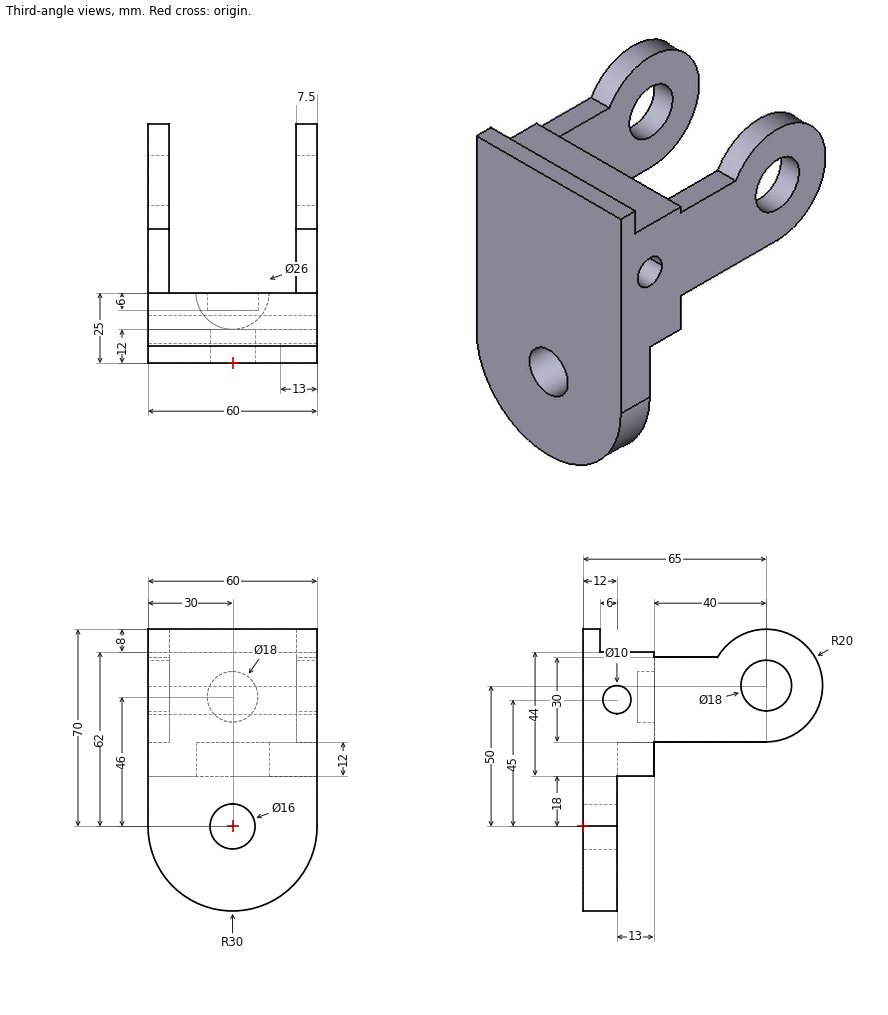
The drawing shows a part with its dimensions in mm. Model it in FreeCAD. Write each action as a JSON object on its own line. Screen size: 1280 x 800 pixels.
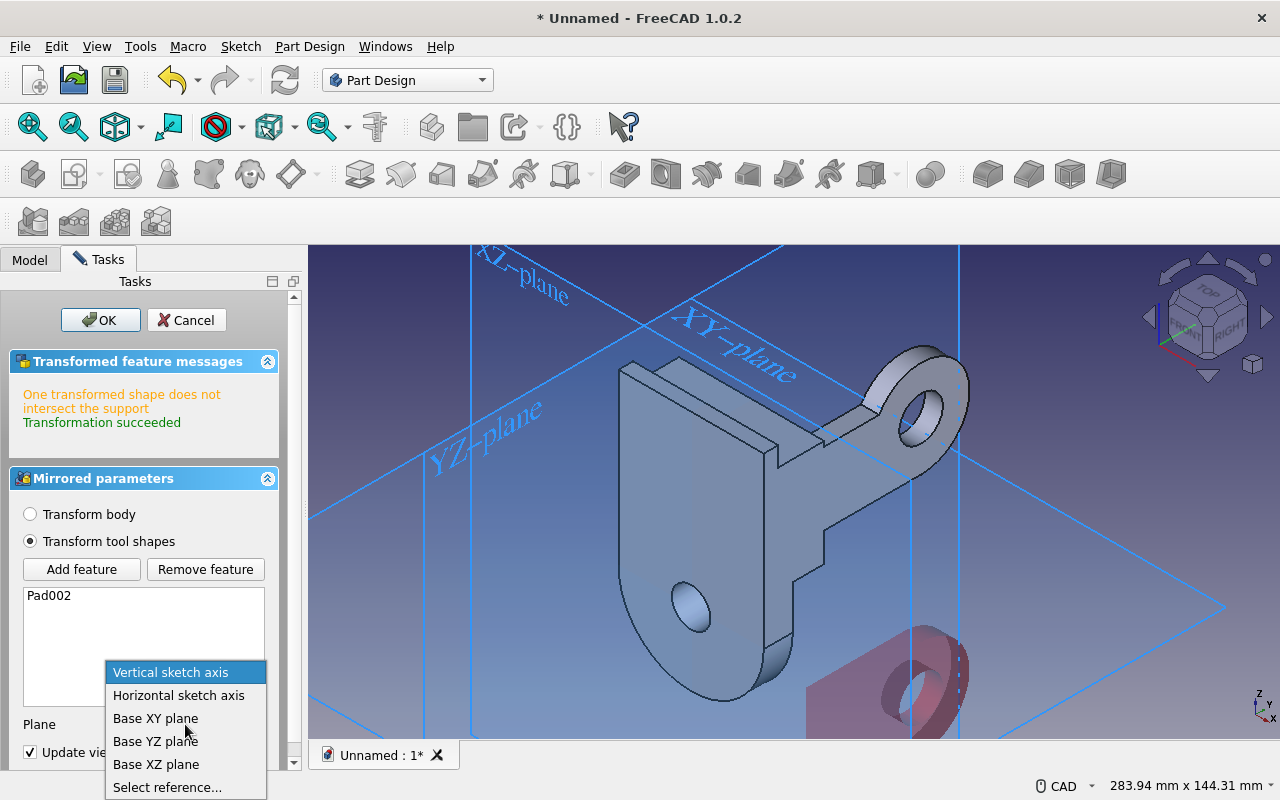
{"action": "left_click", "coordinate": [184, 742]}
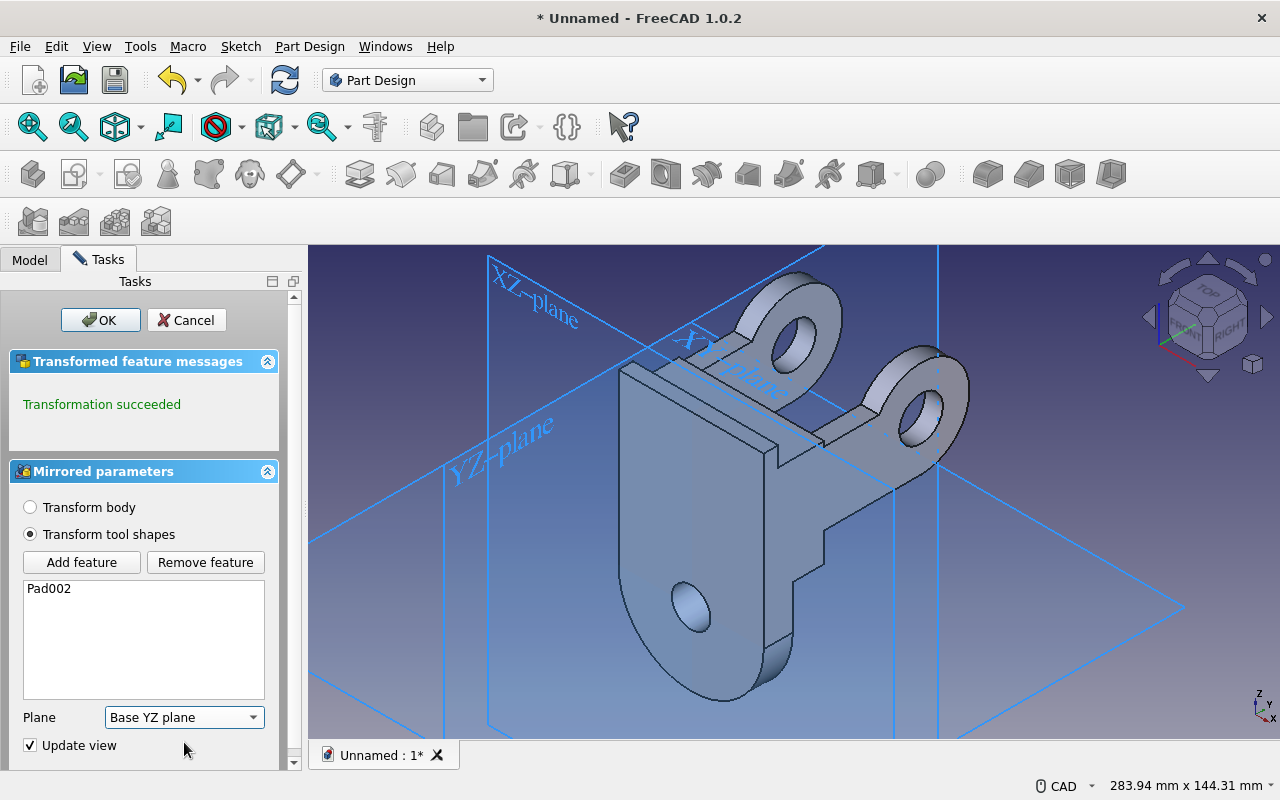
{"action": "left_click", "coordinate": [101, 320]}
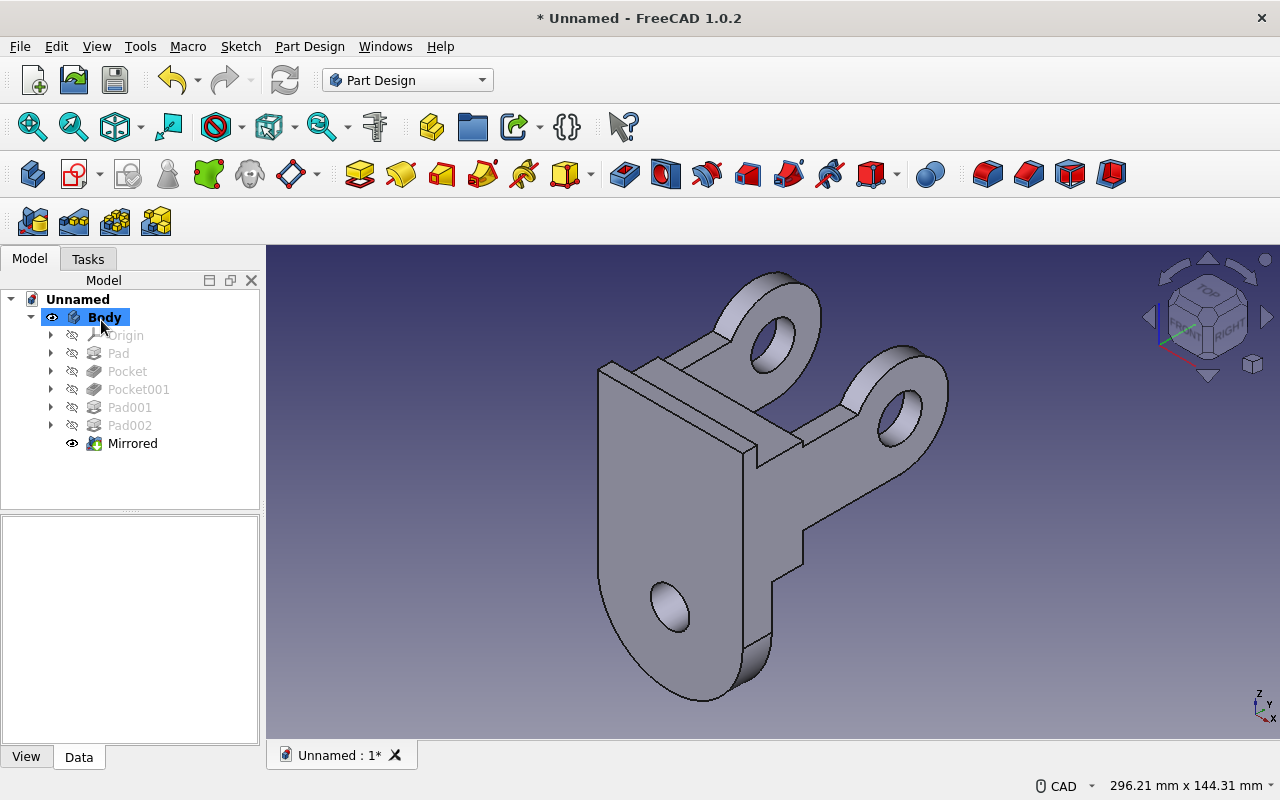
{"action": "key", "text": "5"}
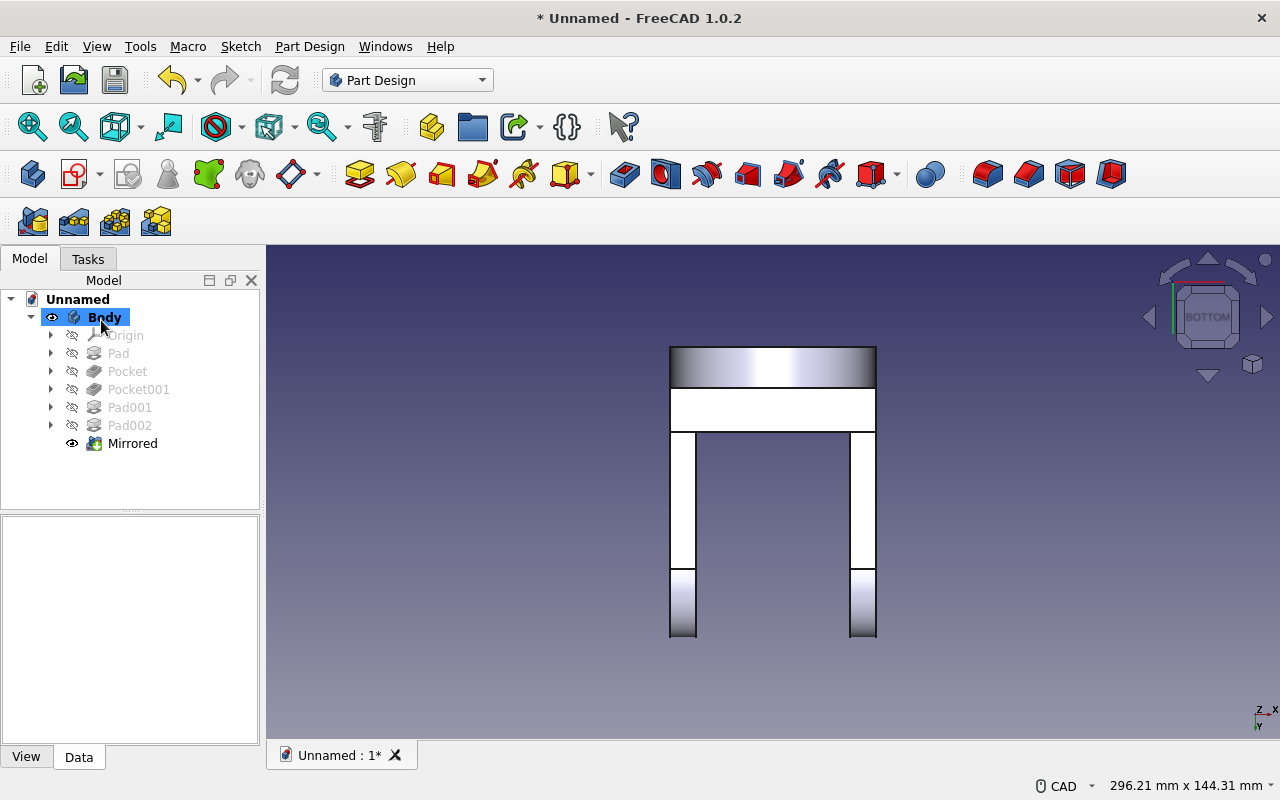
{"action": "left_click", "coordinate": [832, 409]}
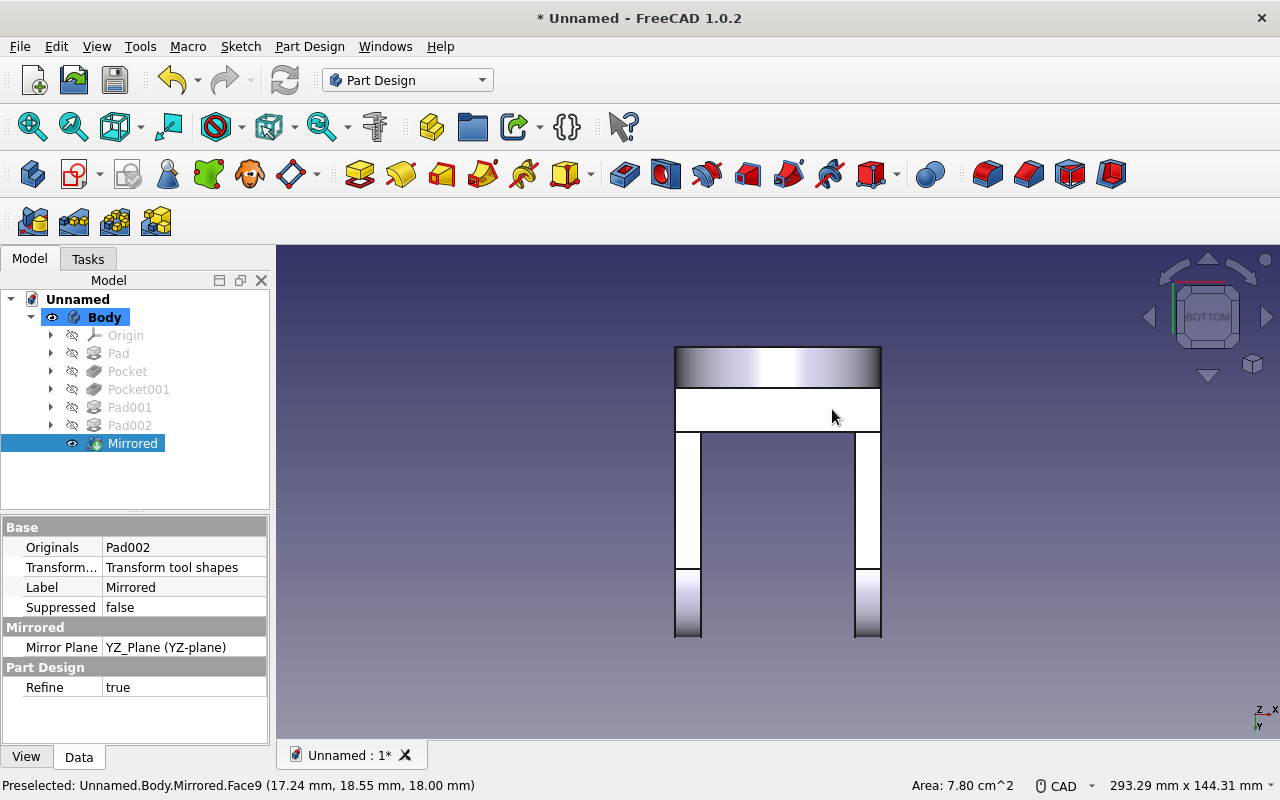
{"action": "left_click", "coordinate": [74, 174]}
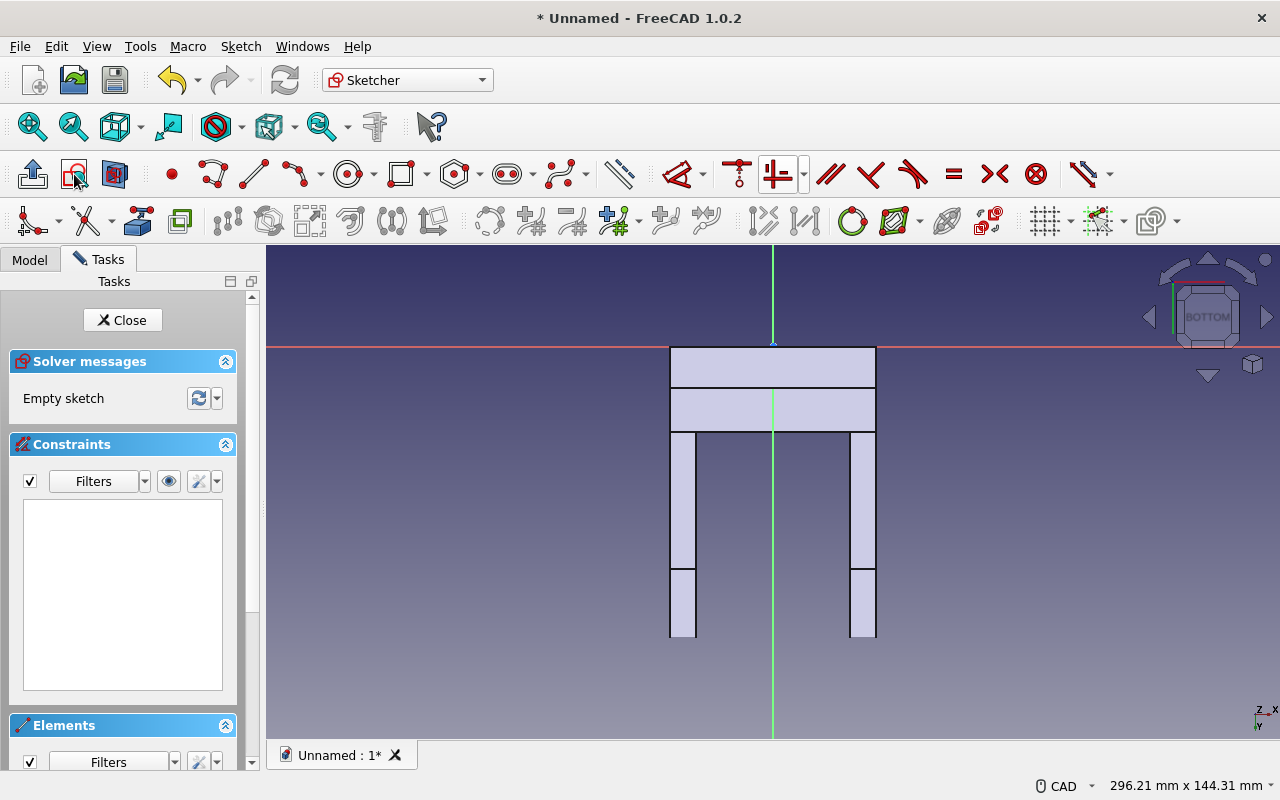
{"action": "scroll", "coordinate": [829, 346], "scroll_direction": "up", "scroll_amount": 4}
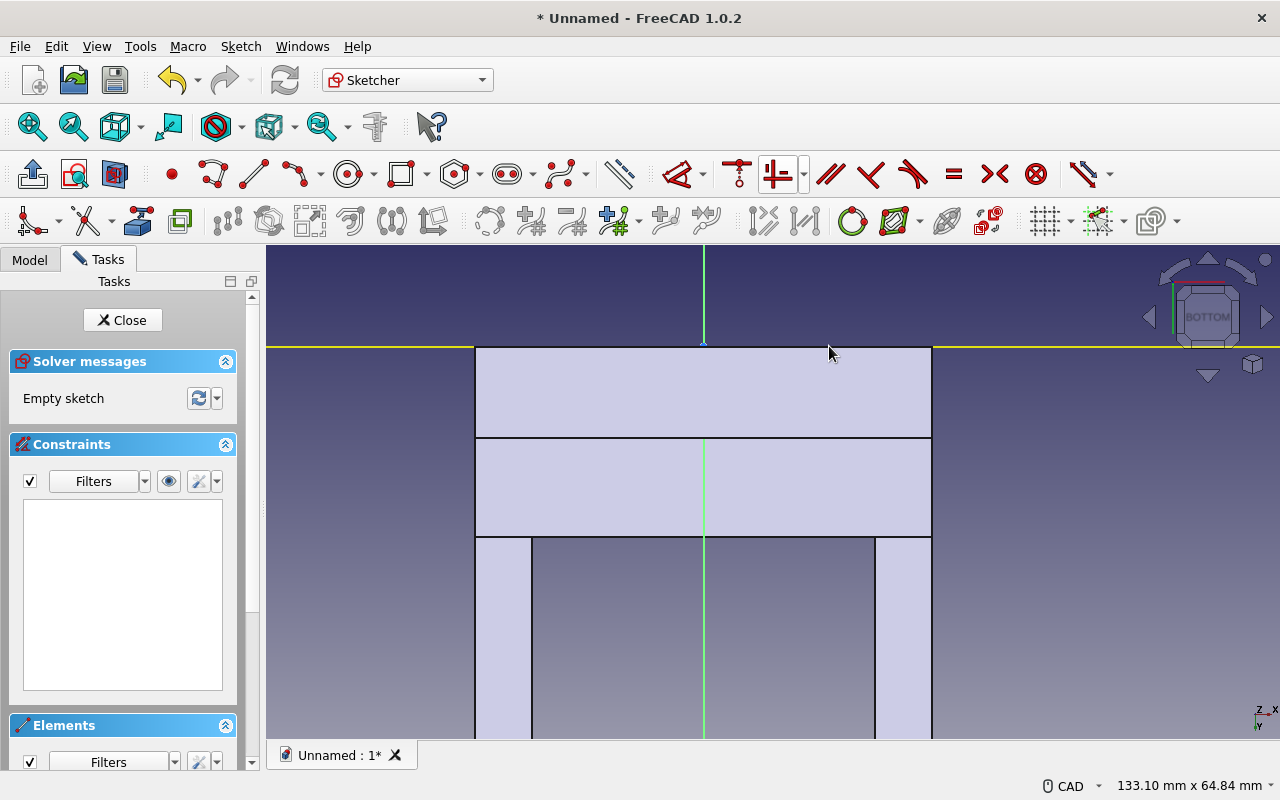
{"action": "key", "text": "g c"}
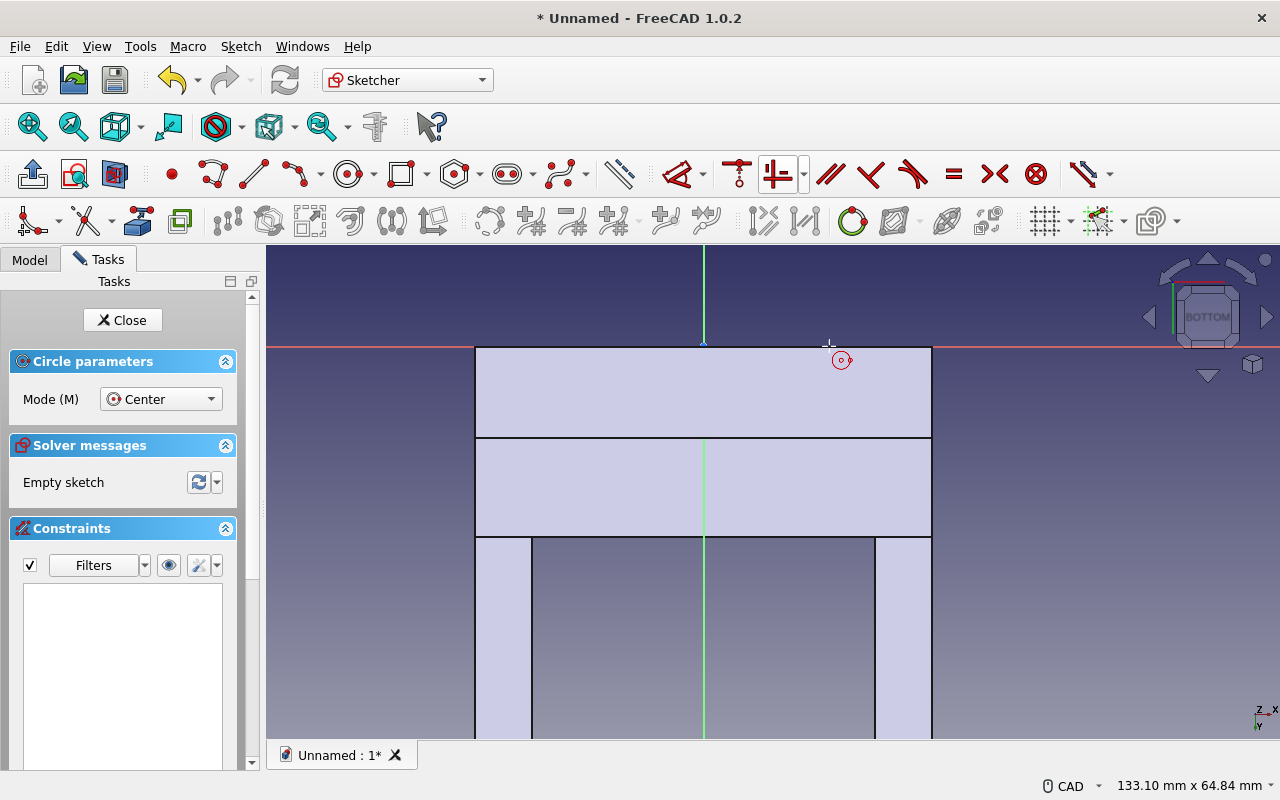
{"action": "left_click", "coordinate": [704, 537]}
{"action": "left_click", "coordinate": [774, 467]}
{"action": "key", "text": "Escape"}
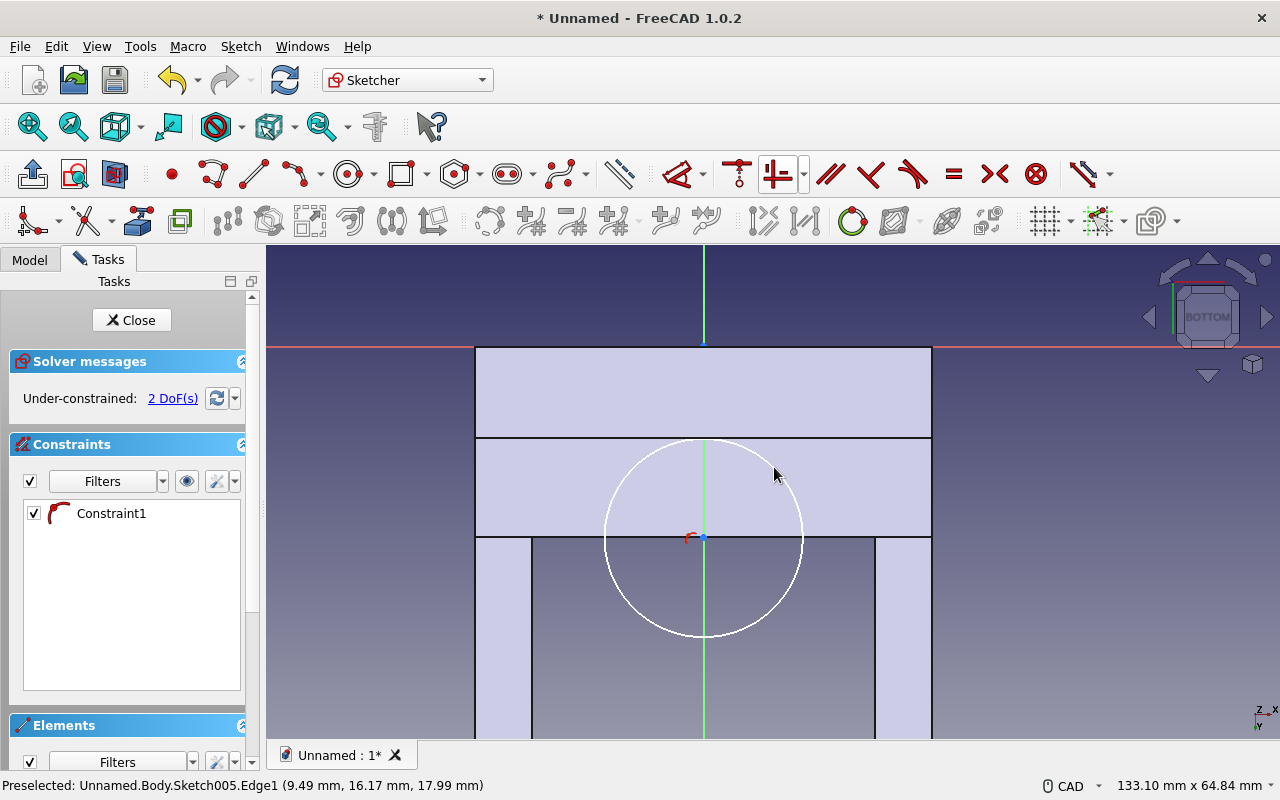
{"action": "key", "text": "d"}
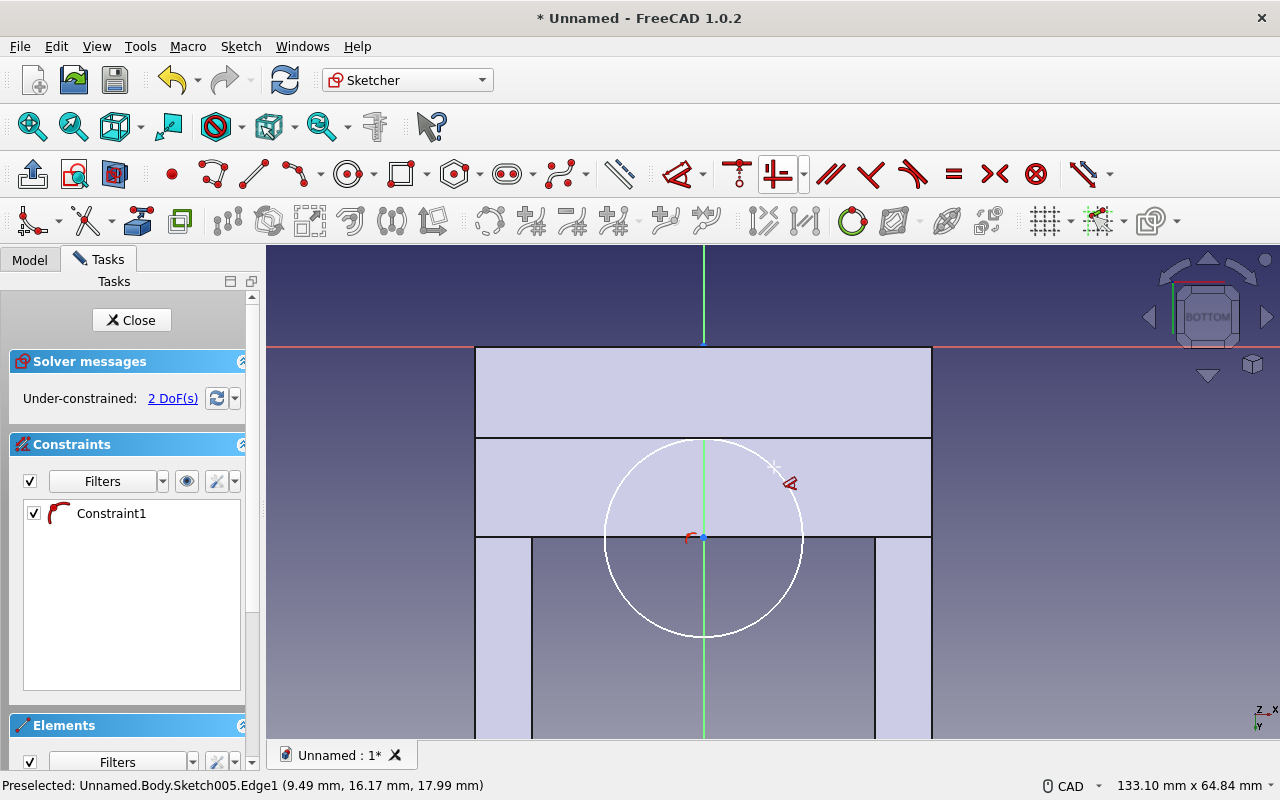
{"action": "left_click", "coordinate": [774, 468]}
{"action": "left_click", "coordinate": [797, 445]}